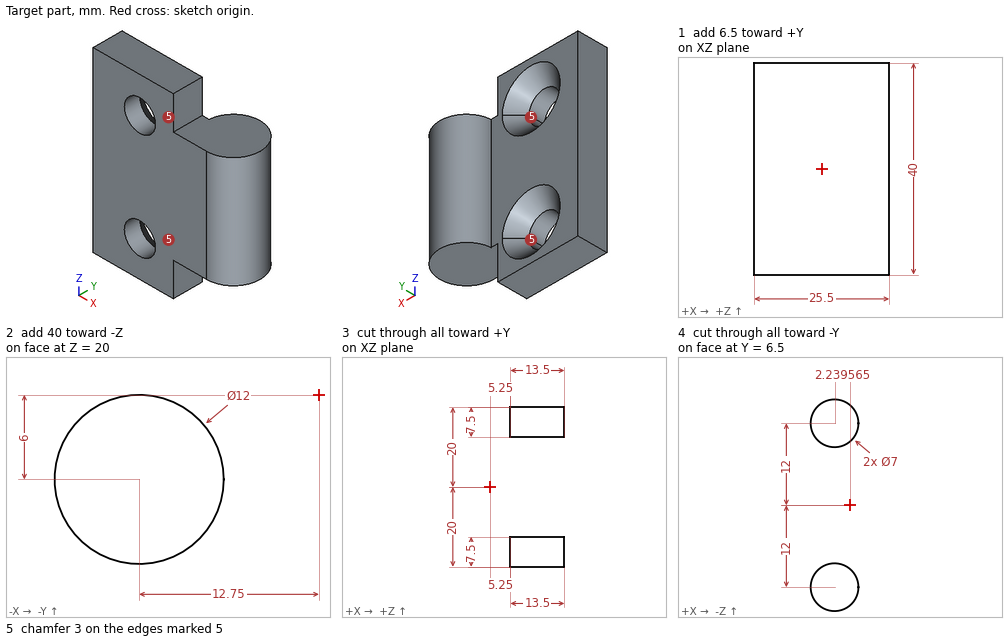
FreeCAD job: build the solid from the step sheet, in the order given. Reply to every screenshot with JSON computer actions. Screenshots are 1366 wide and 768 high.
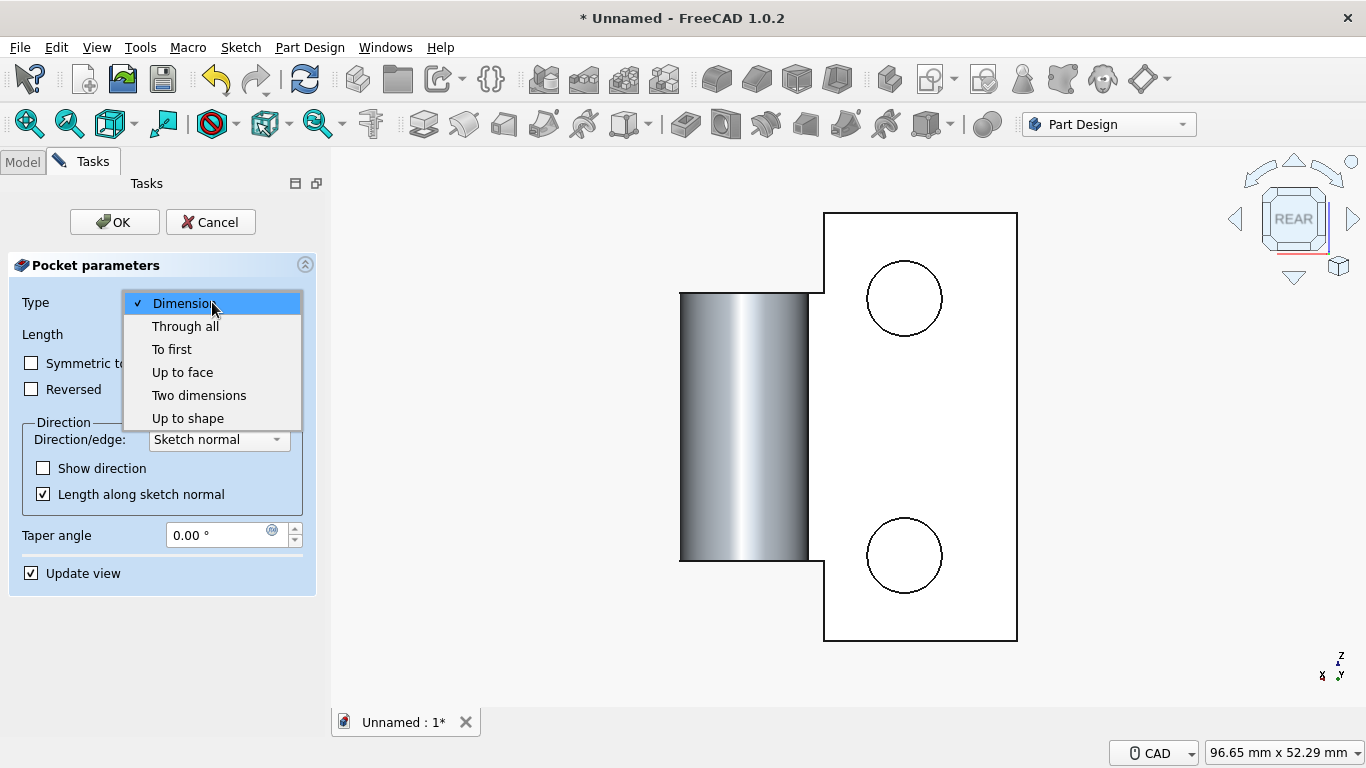
{"action": "left_click", "coordinate": [212, 326]}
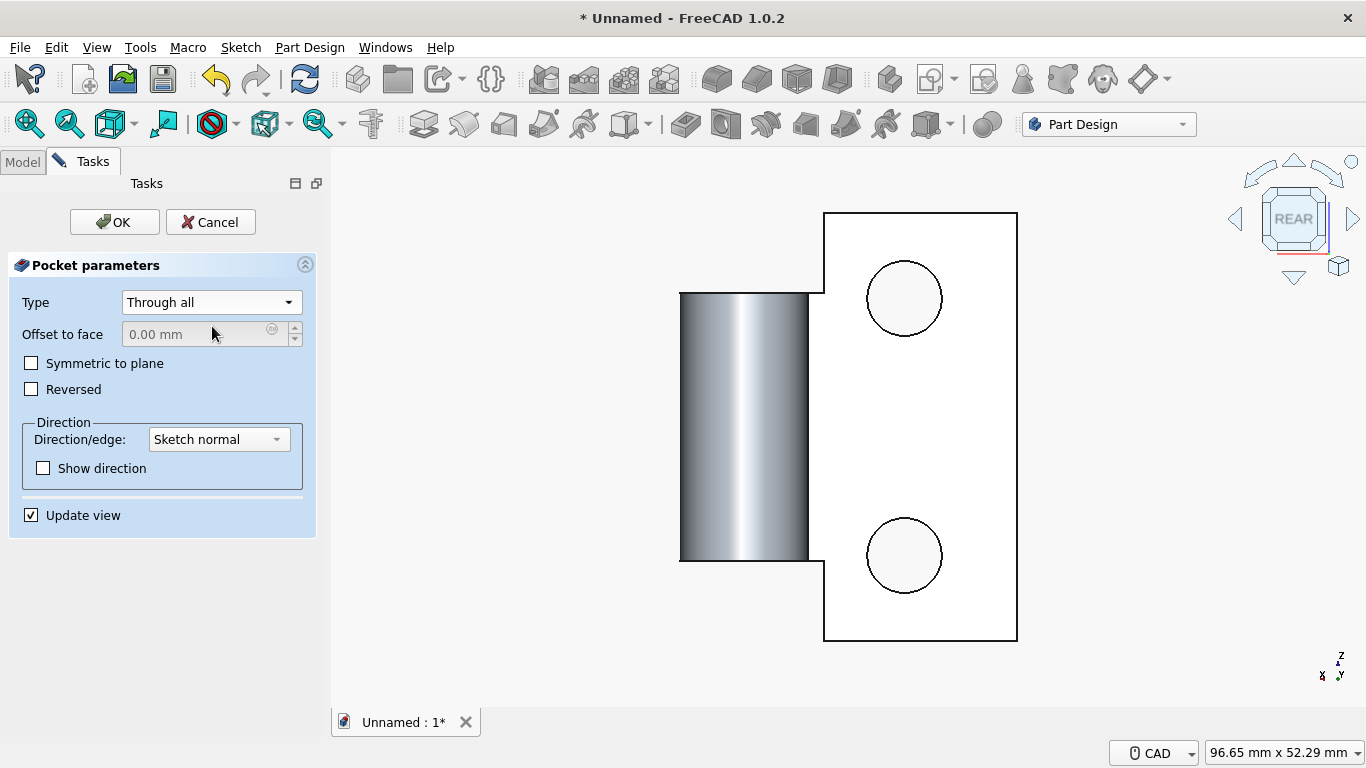
{"action": "left_click", "coordinate": [115, 222]}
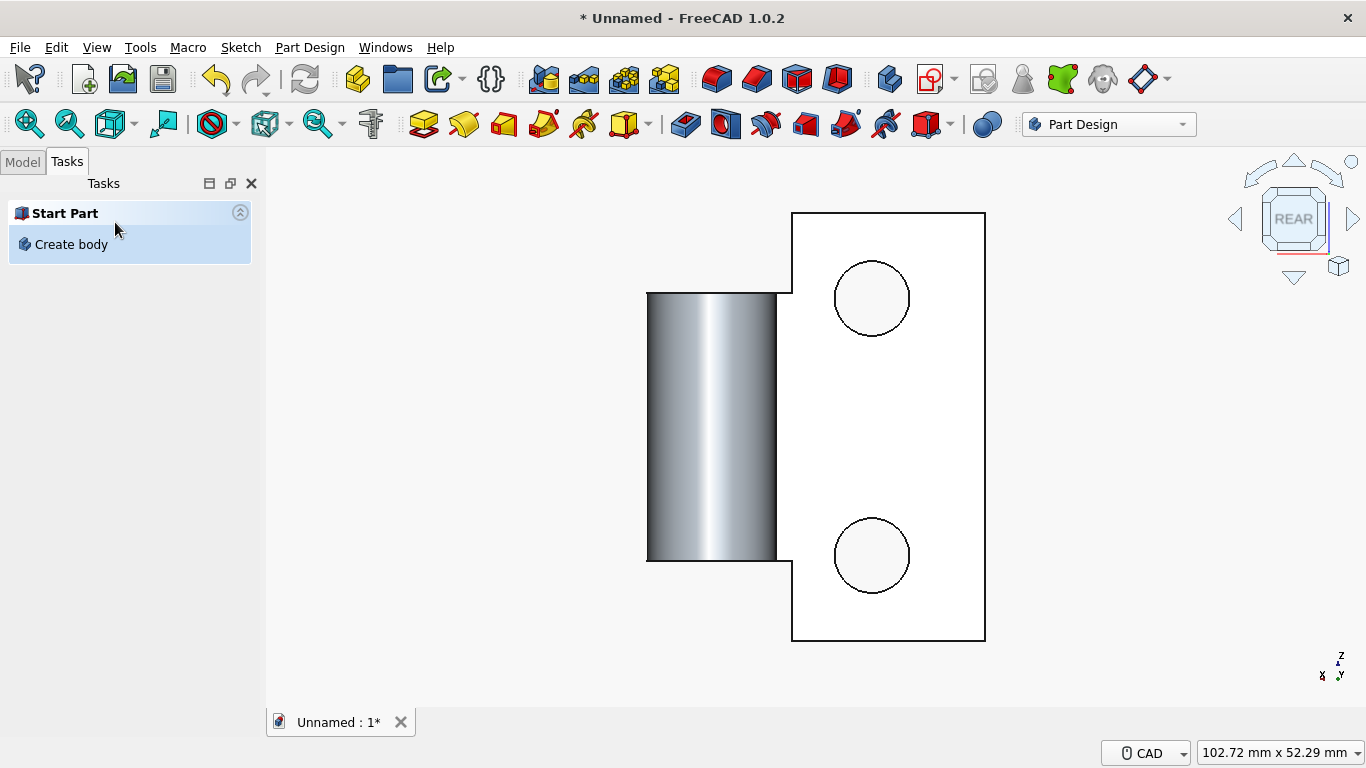
{"action": "left_click", "coordinate": [902, 533]}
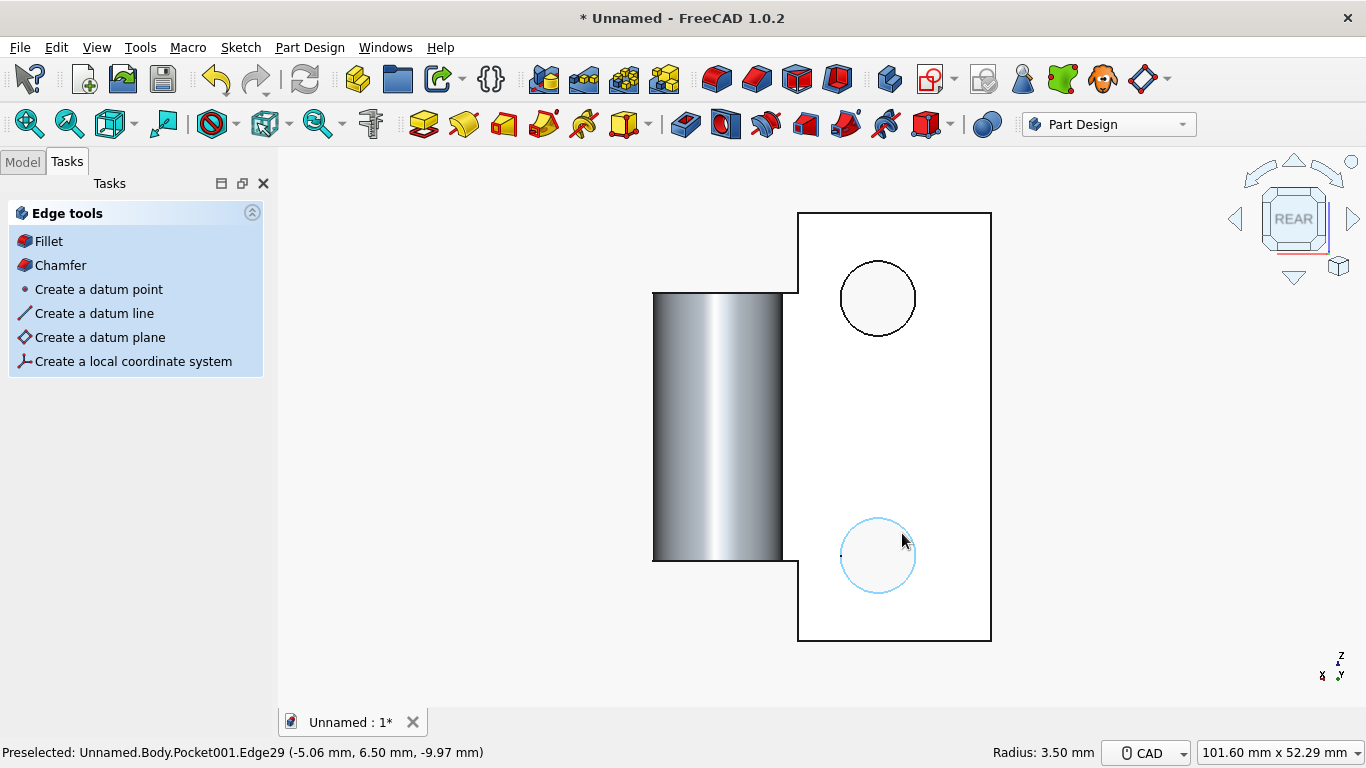
{"action": "left_click", "coordinate": [908, 276], "text": "ctrl"}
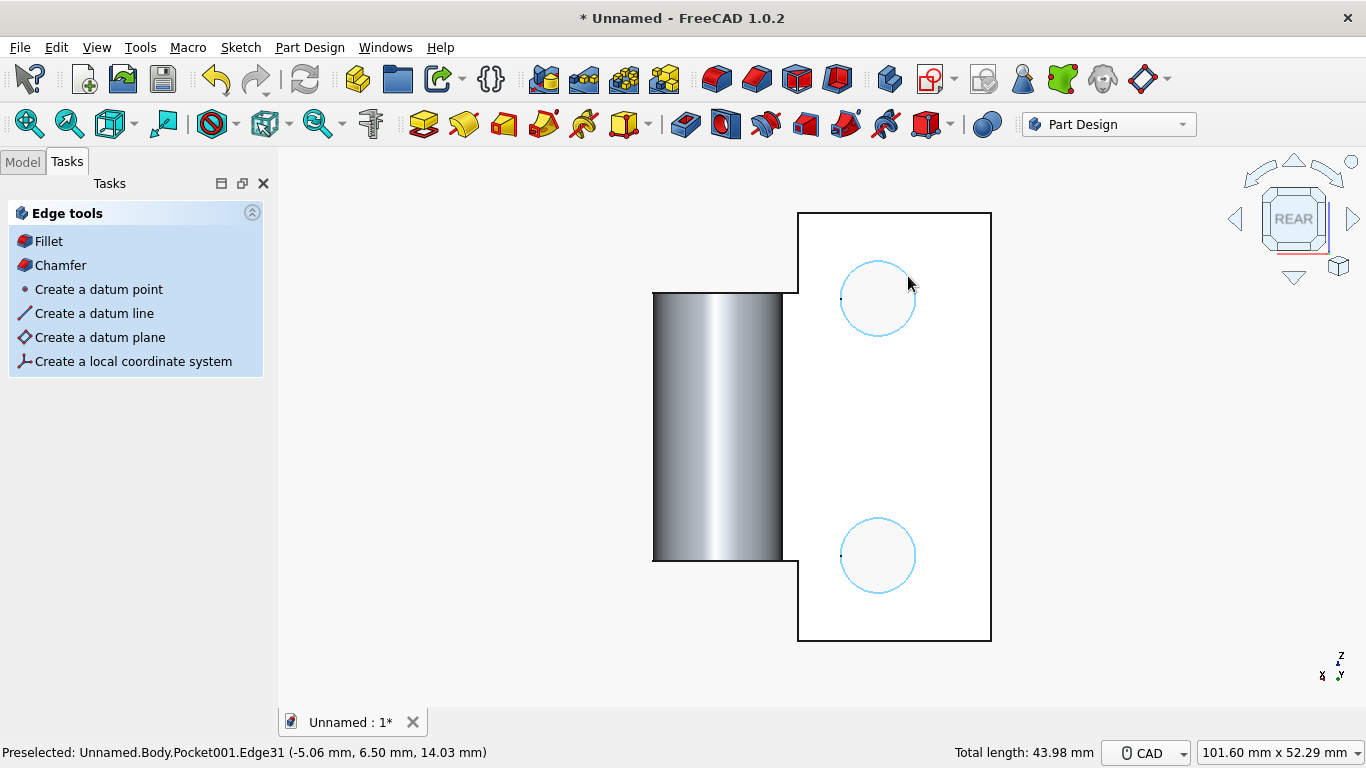
{"action": "left_click", "coordinate": [758, 80]}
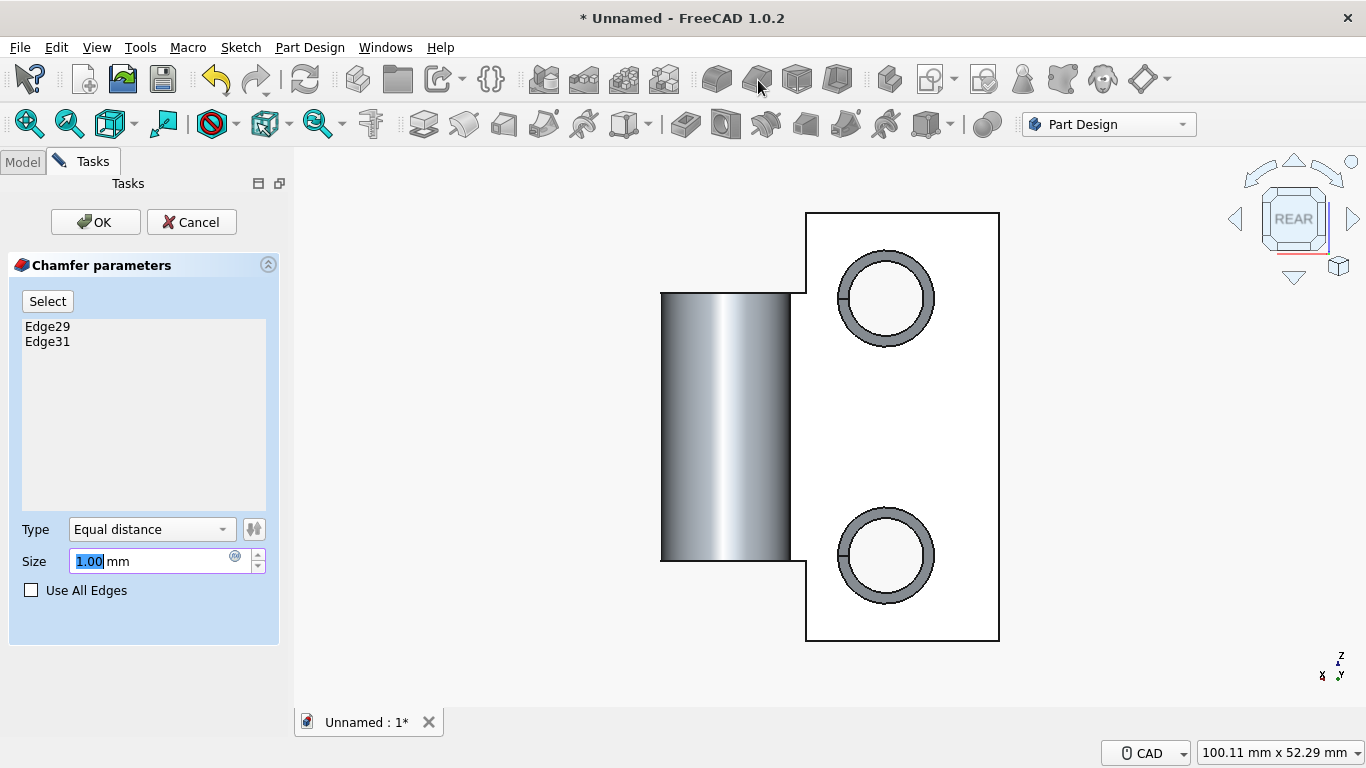
{"action": "type", "text": "3"}
{"action": "key", "text": "Tab"}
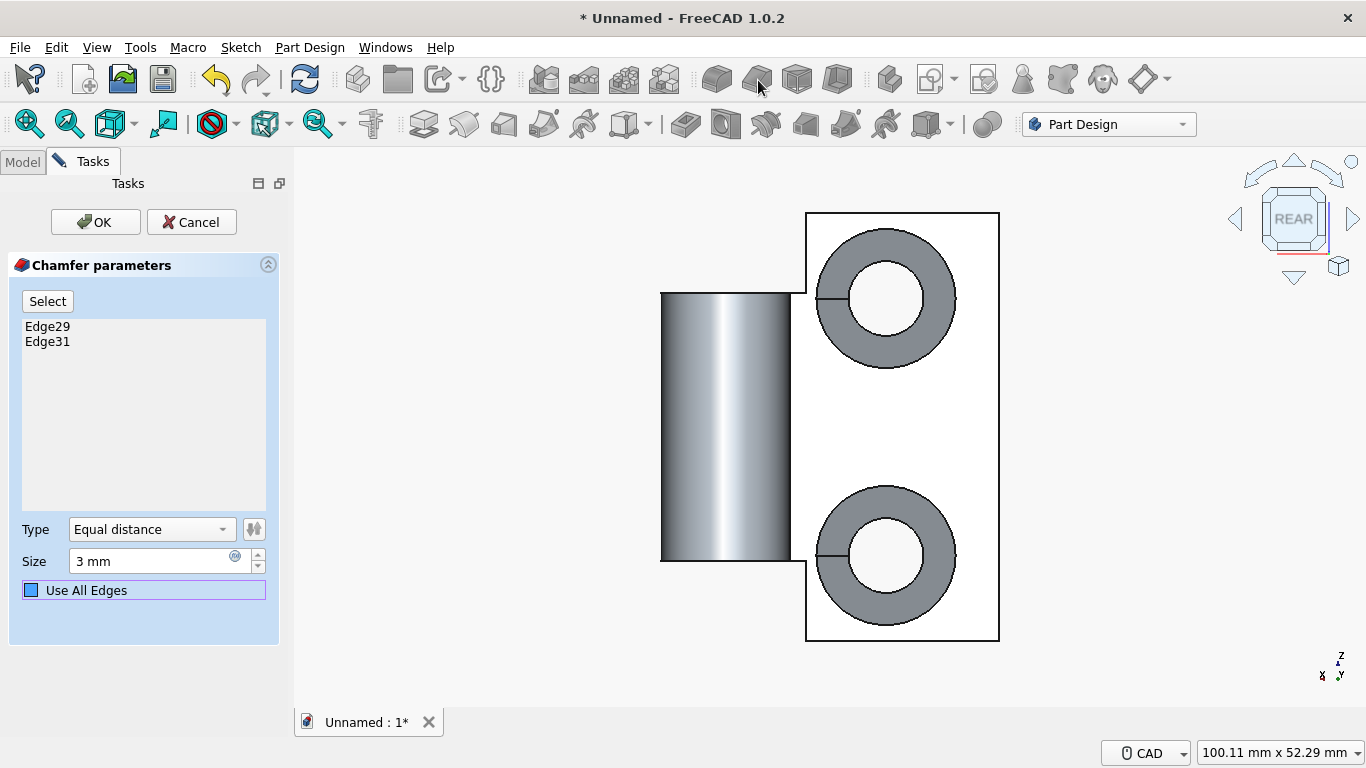
{"action": "left_click", "coordinate": [96, 222]}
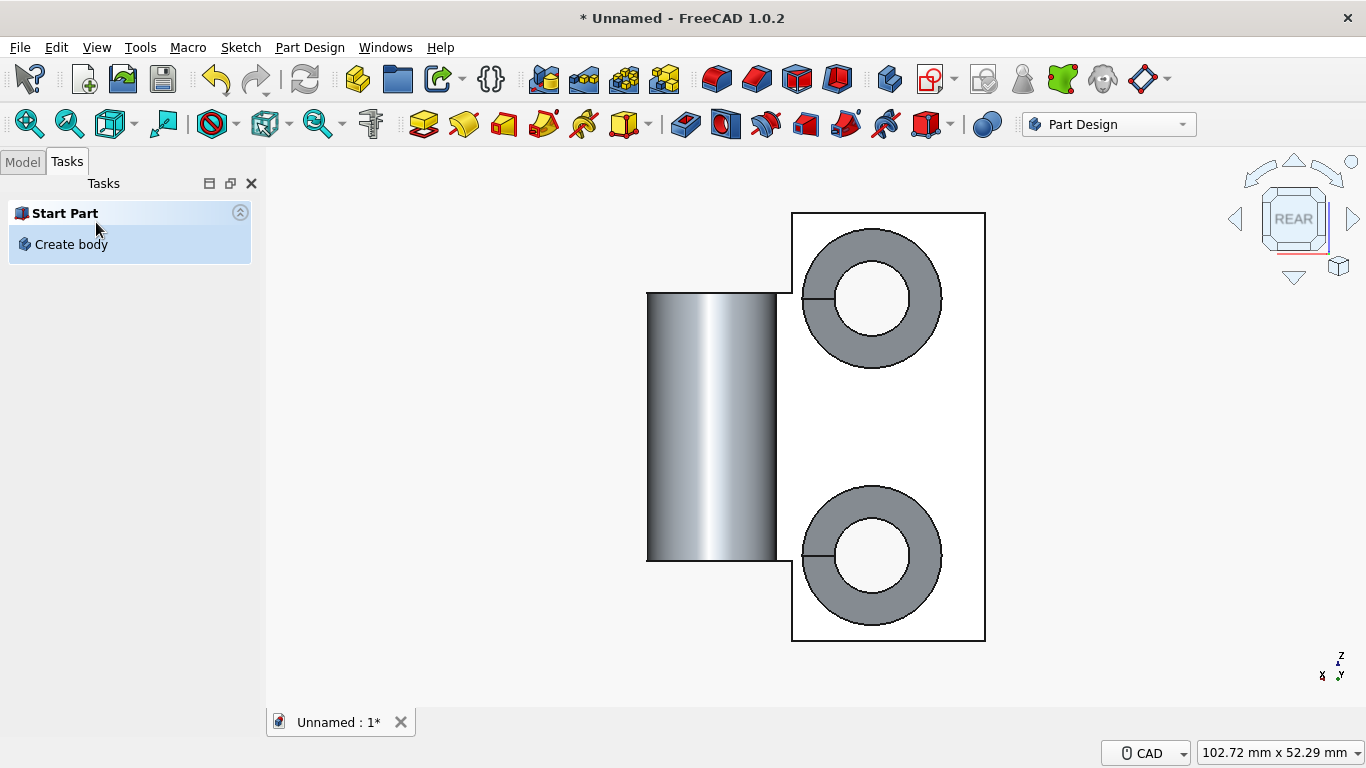
{"action": "key", "text": "0"}